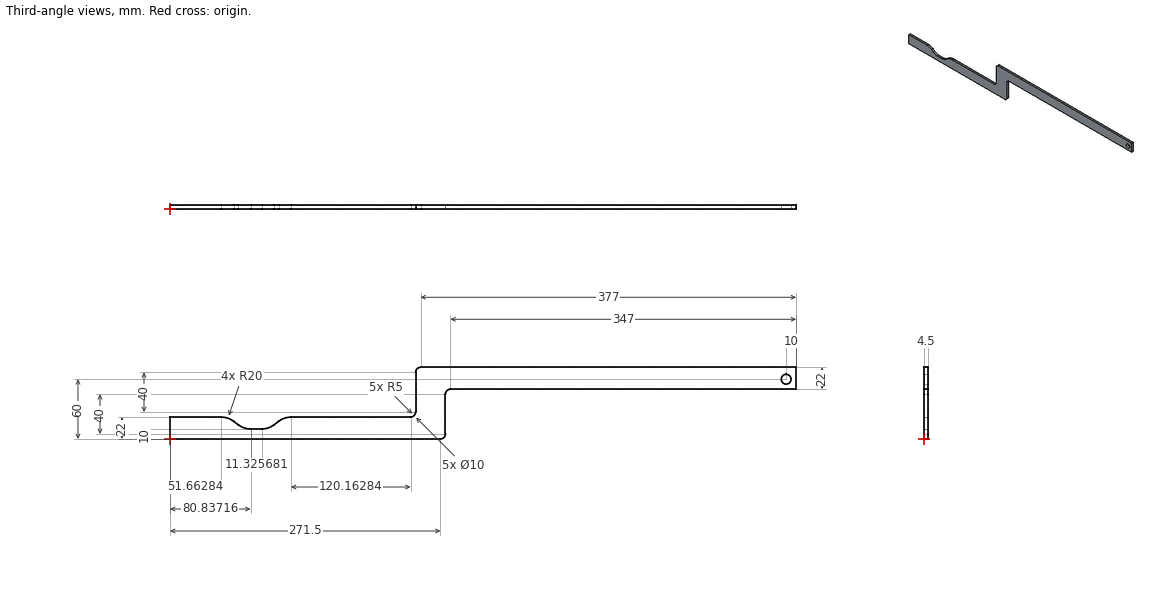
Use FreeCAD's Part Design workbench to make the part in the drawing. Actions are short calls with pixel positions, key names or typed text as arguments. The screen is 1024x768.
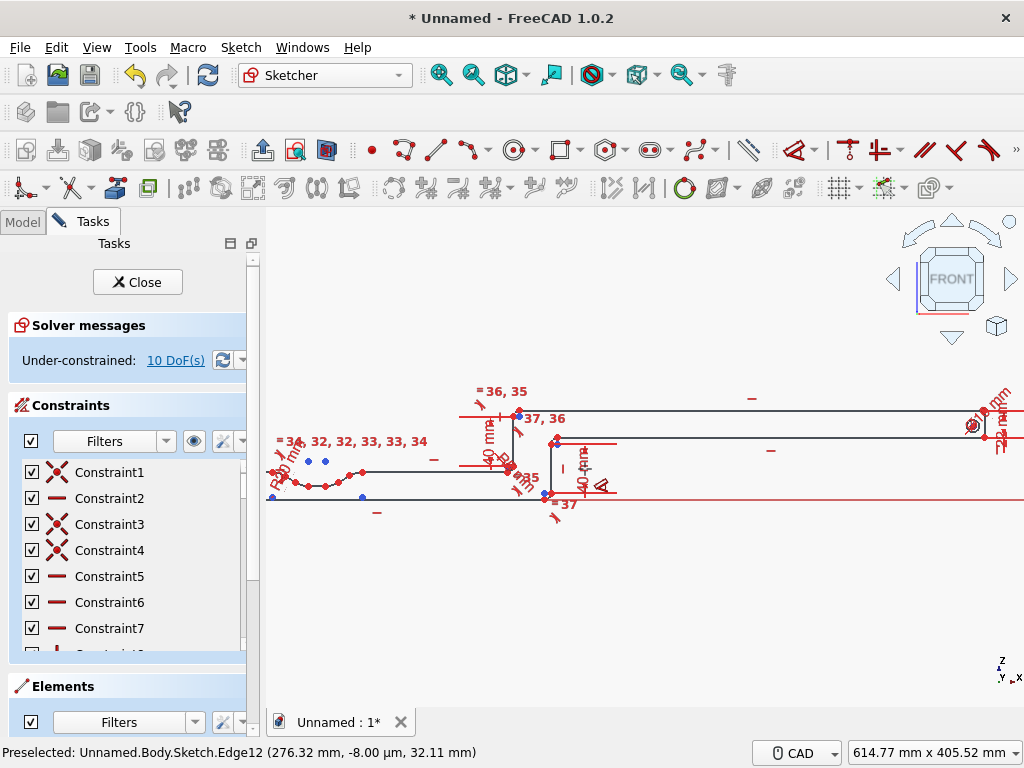
scroll(551, 459, down, 3)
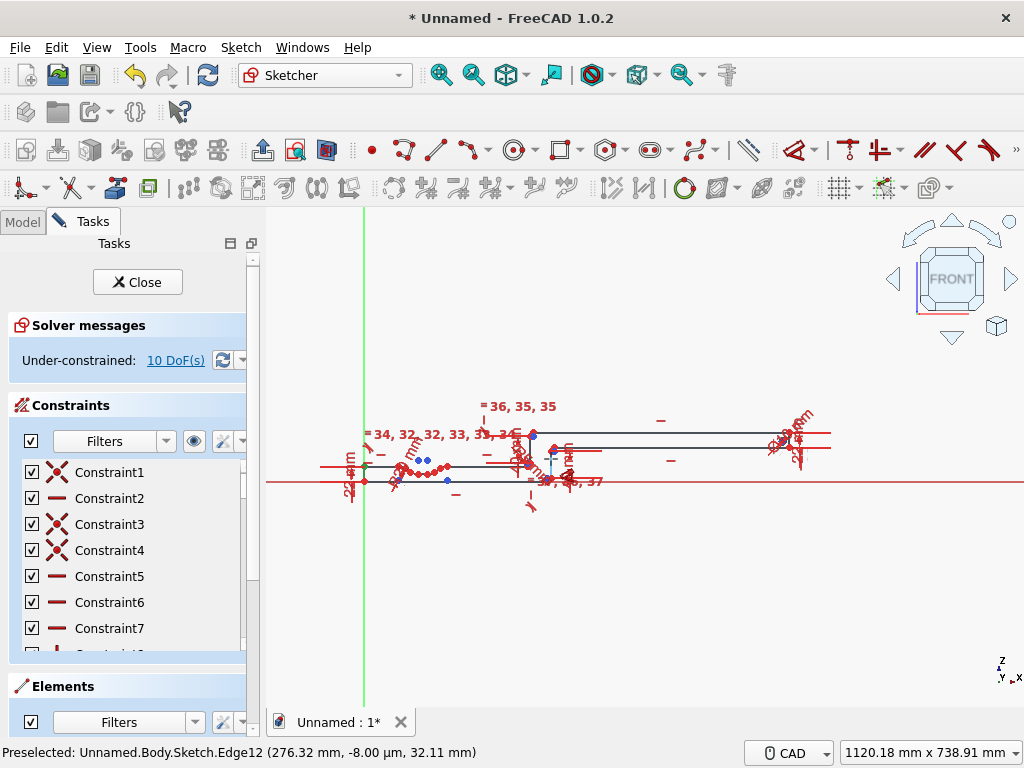
scroll(783, 441, up, 2)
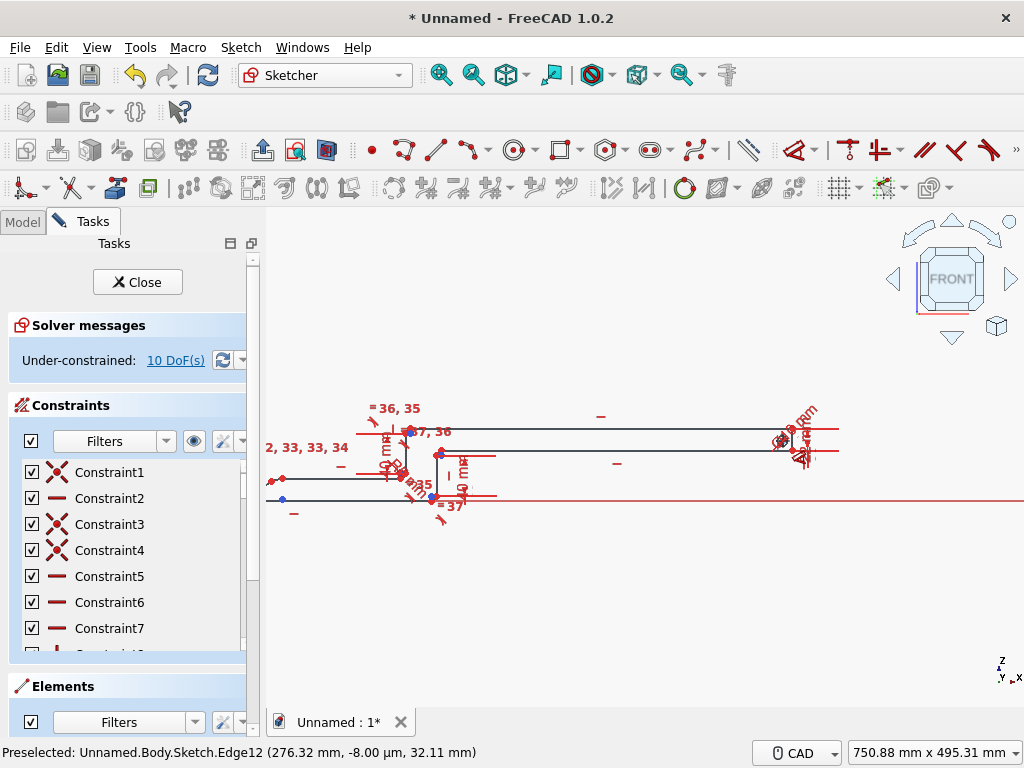
click(782, 441)
click(816, 471)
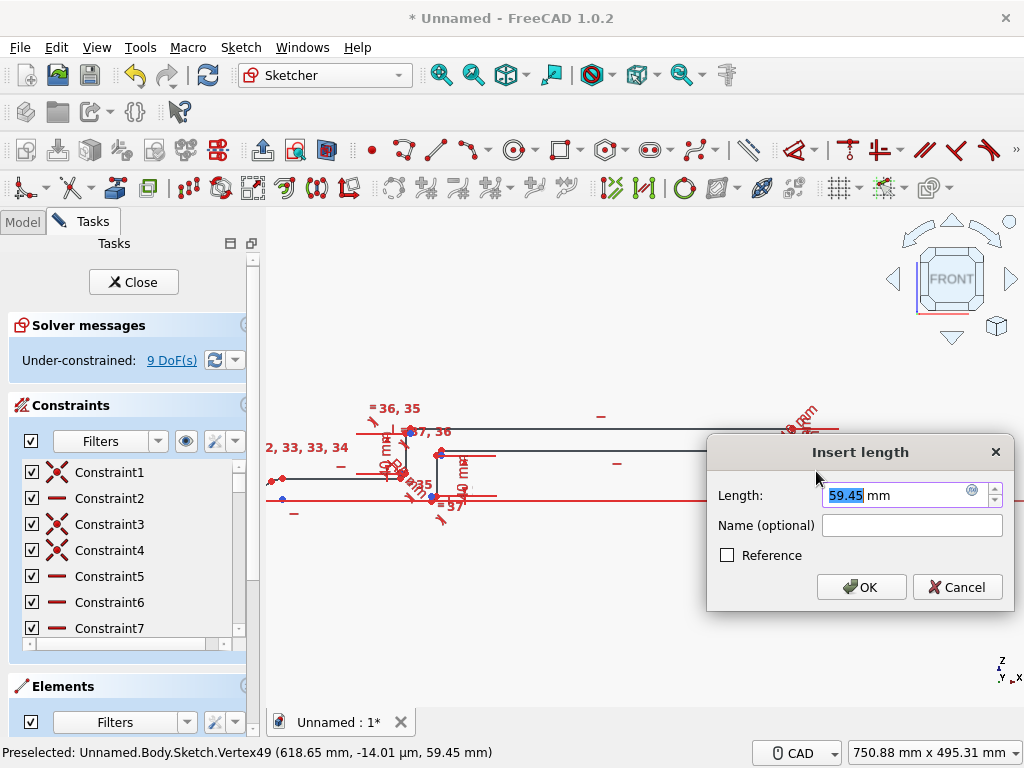
text(60)
key(Return)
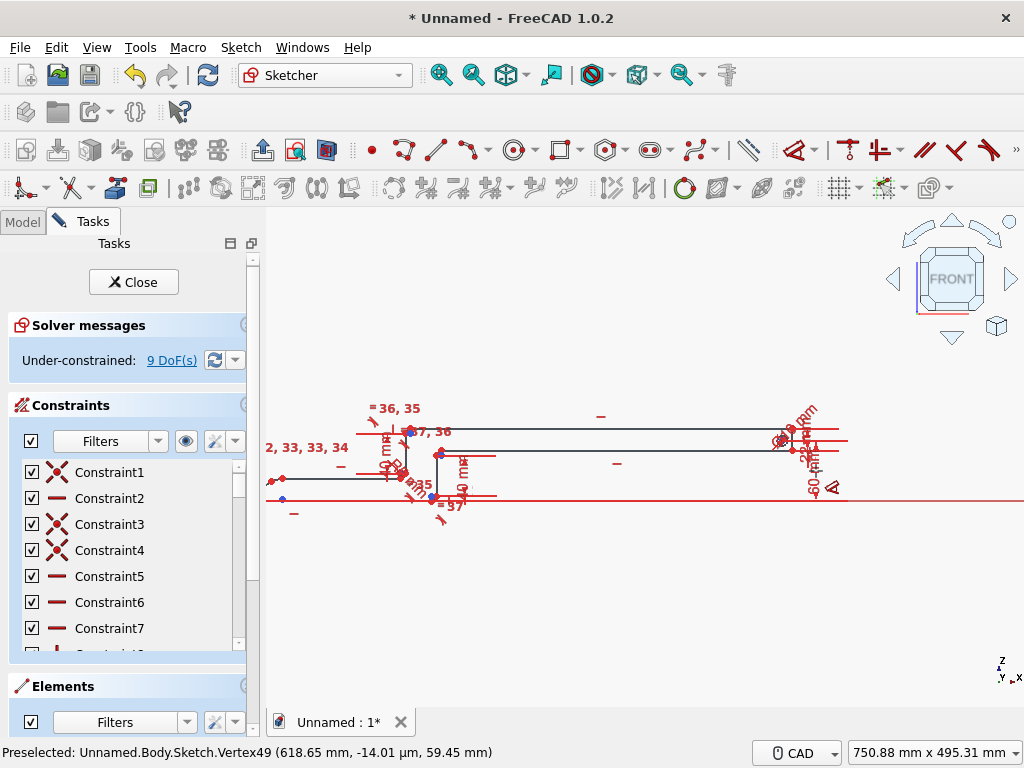
click(525, 429)
click(602, 395)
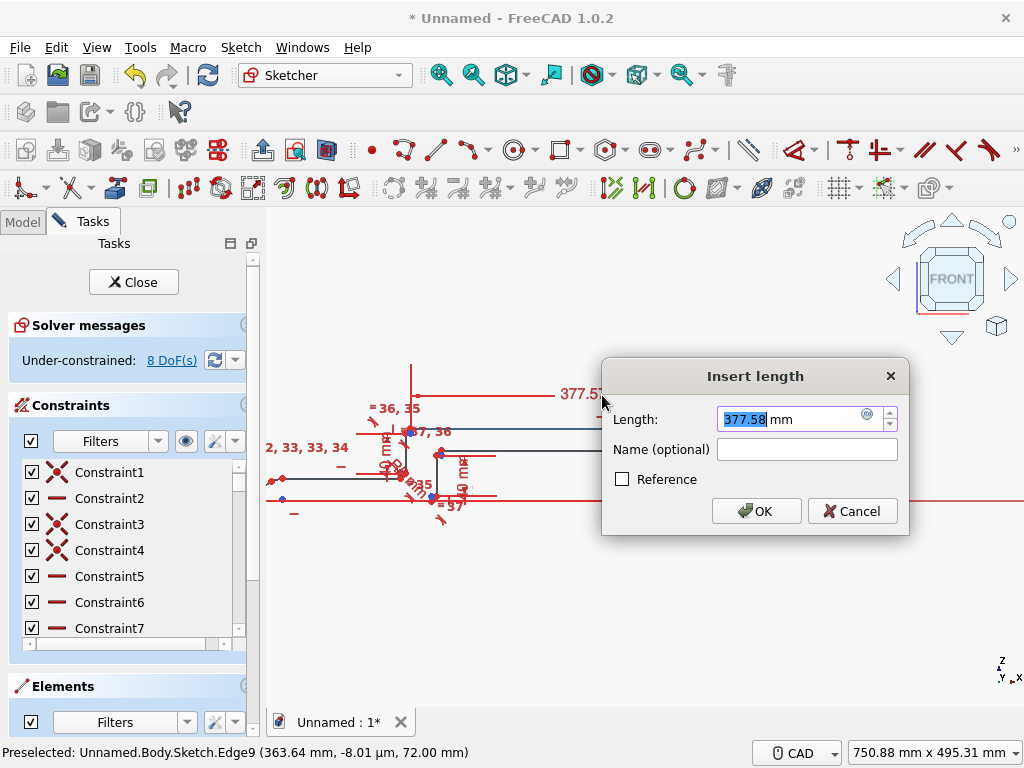
text(377)
key(Return)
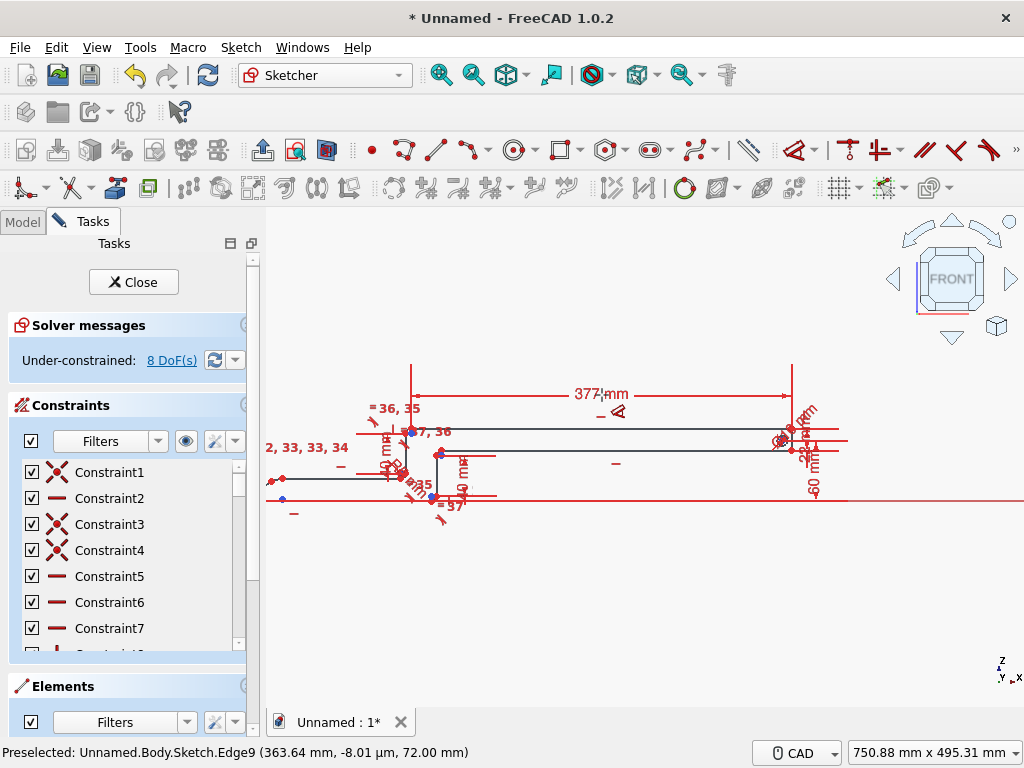
click(687, 451)
click(617, 485)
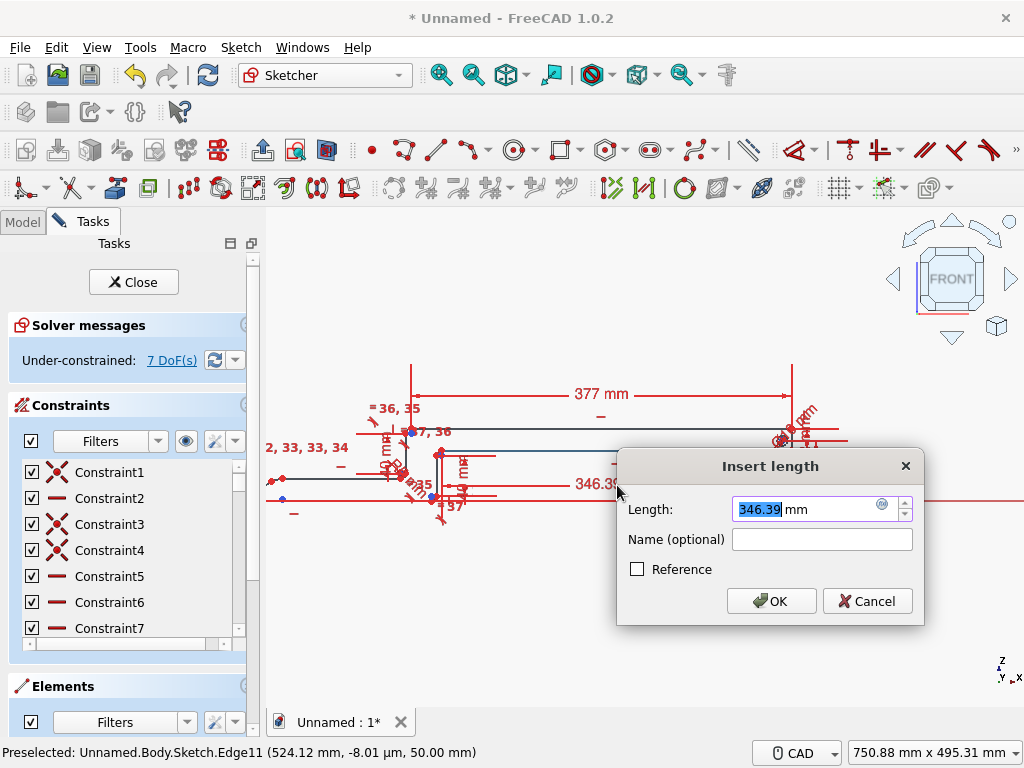
text(347)
key(Return)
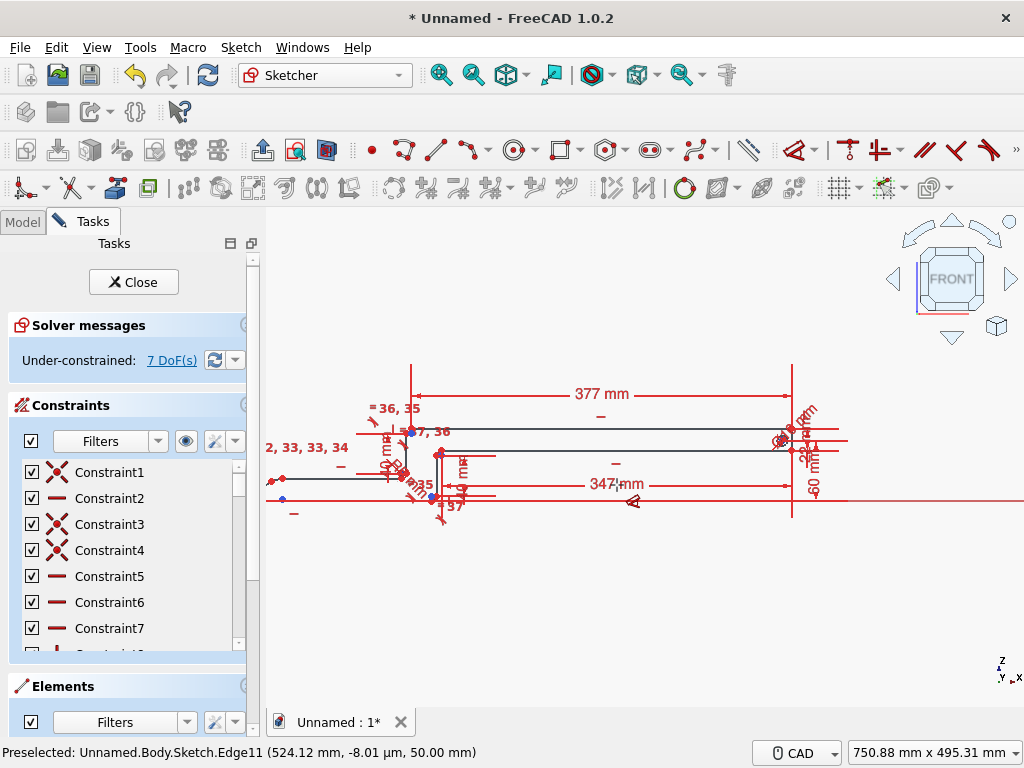
scroll(783, 441, down, 2)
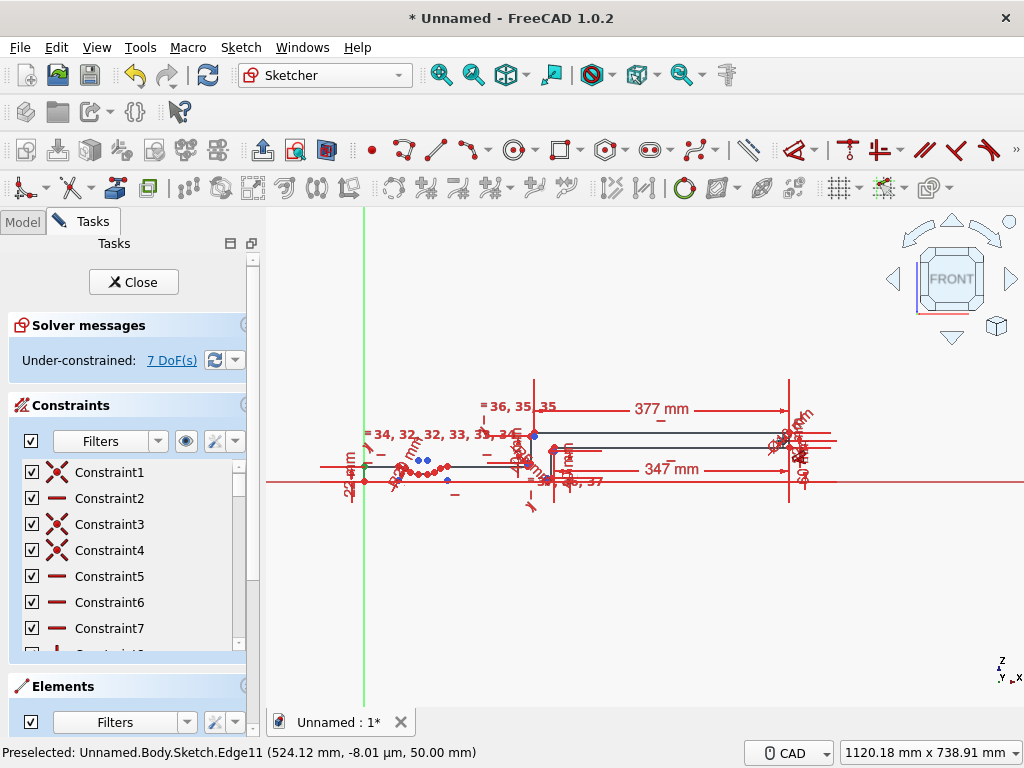
scroll(418, 474, up, 9)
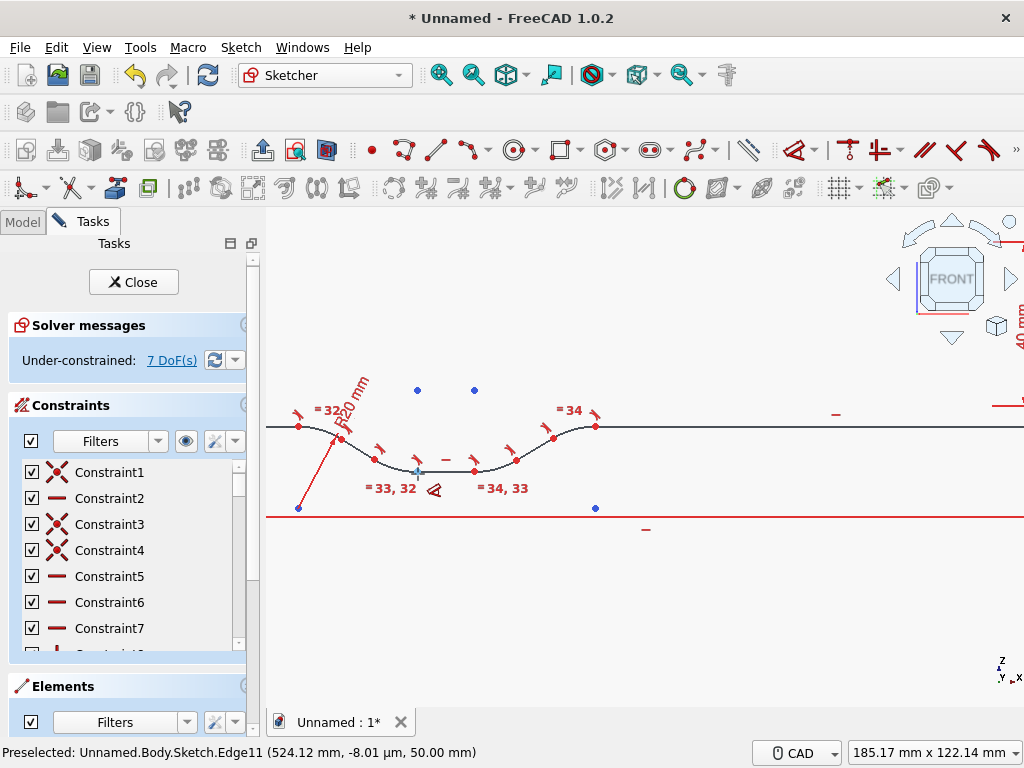
click(417, 472)
click(451, 494)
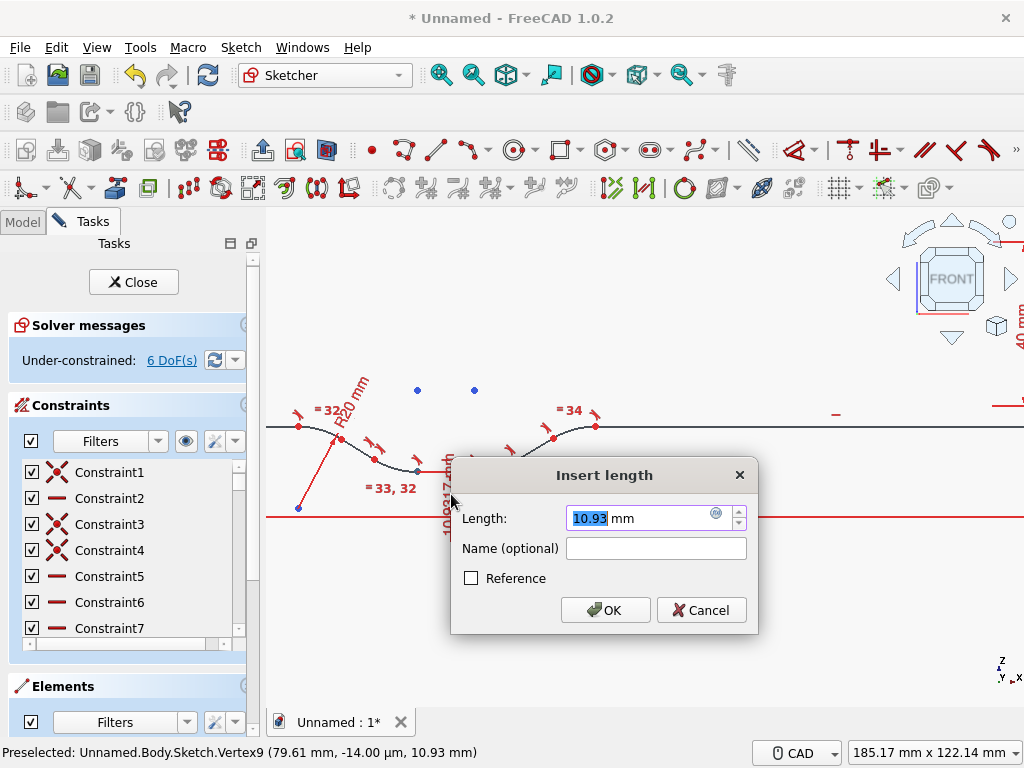
text(10)
key(Return)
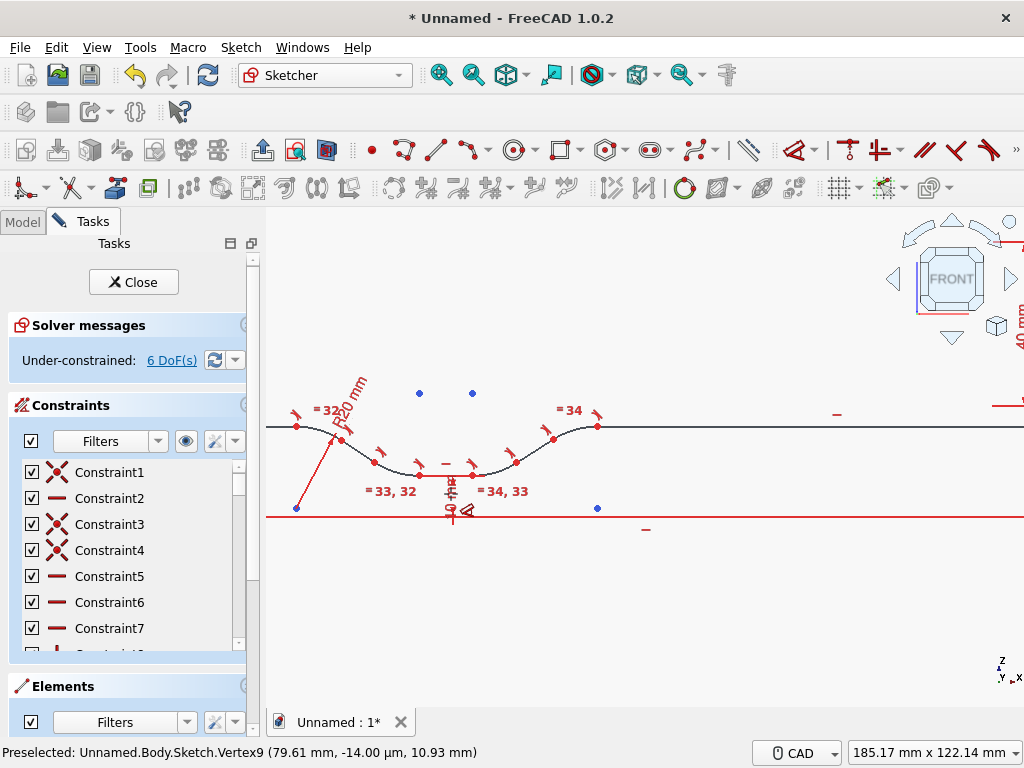
scroll(418, 474, down, 9)